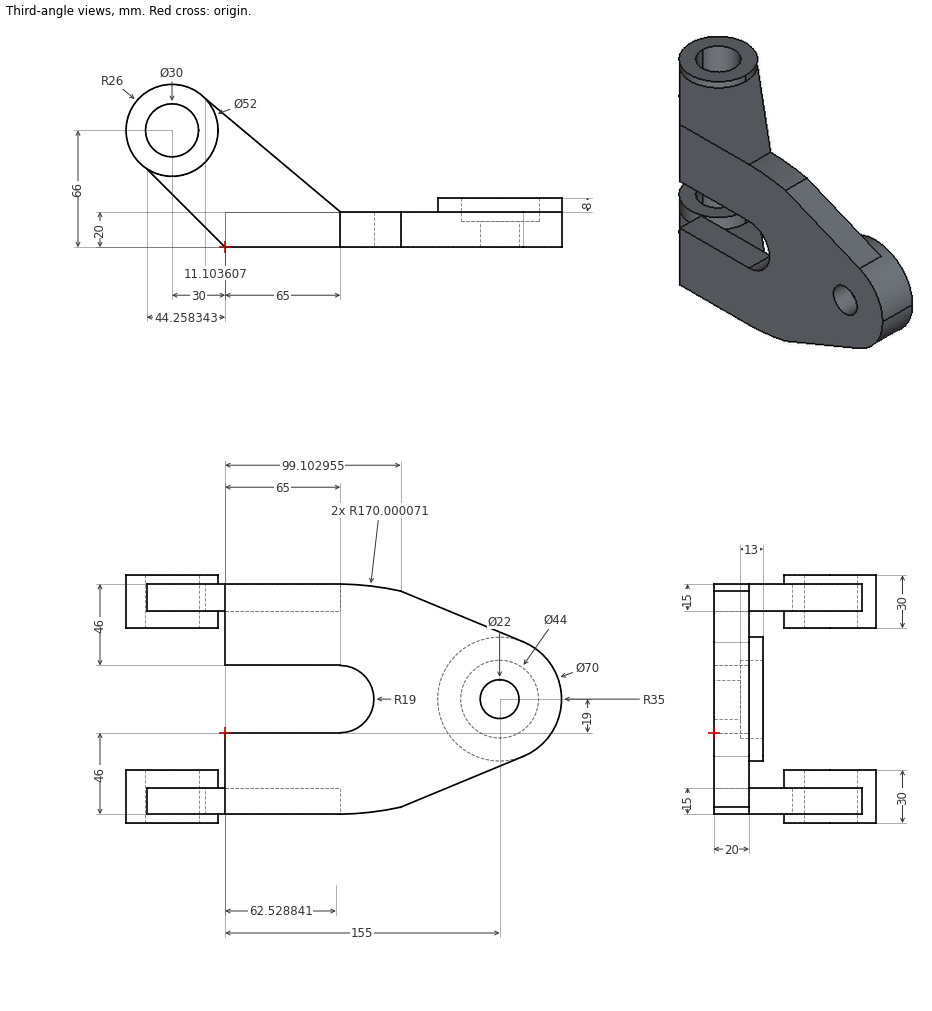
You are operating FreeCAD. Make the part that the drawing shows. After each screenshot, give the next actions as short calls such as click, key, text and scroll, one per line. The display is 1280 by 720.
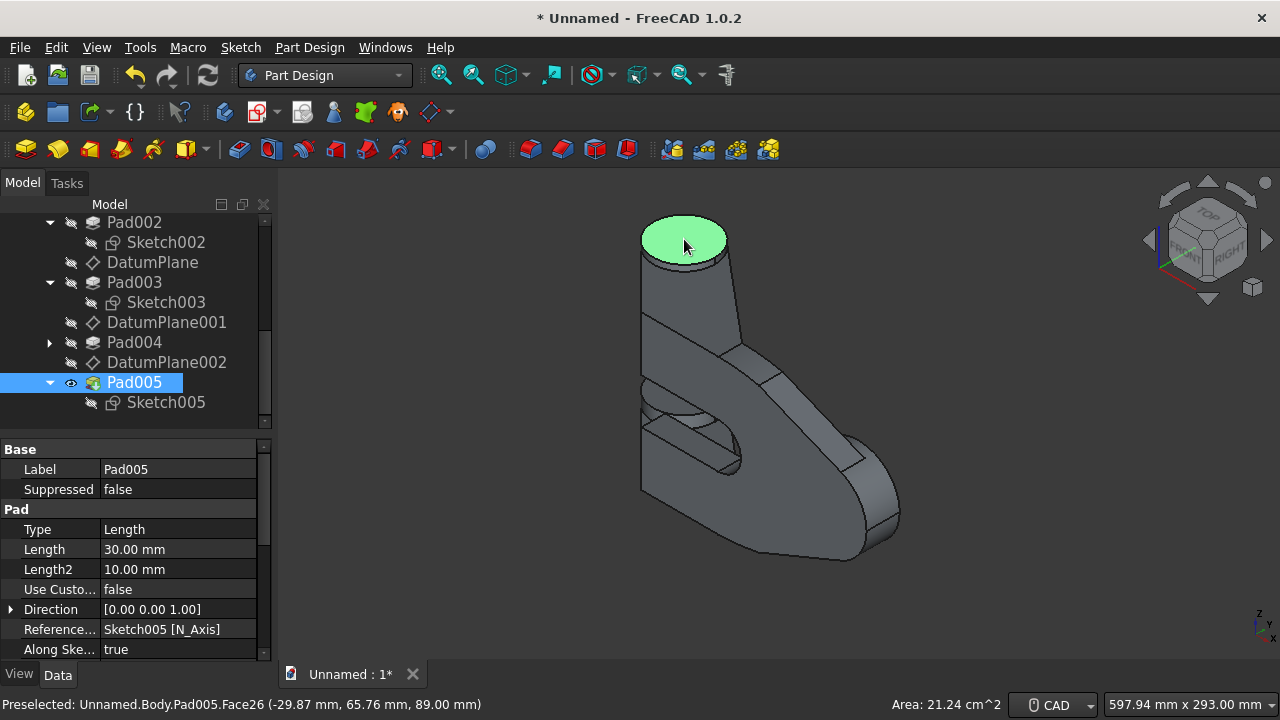
click(258, 112)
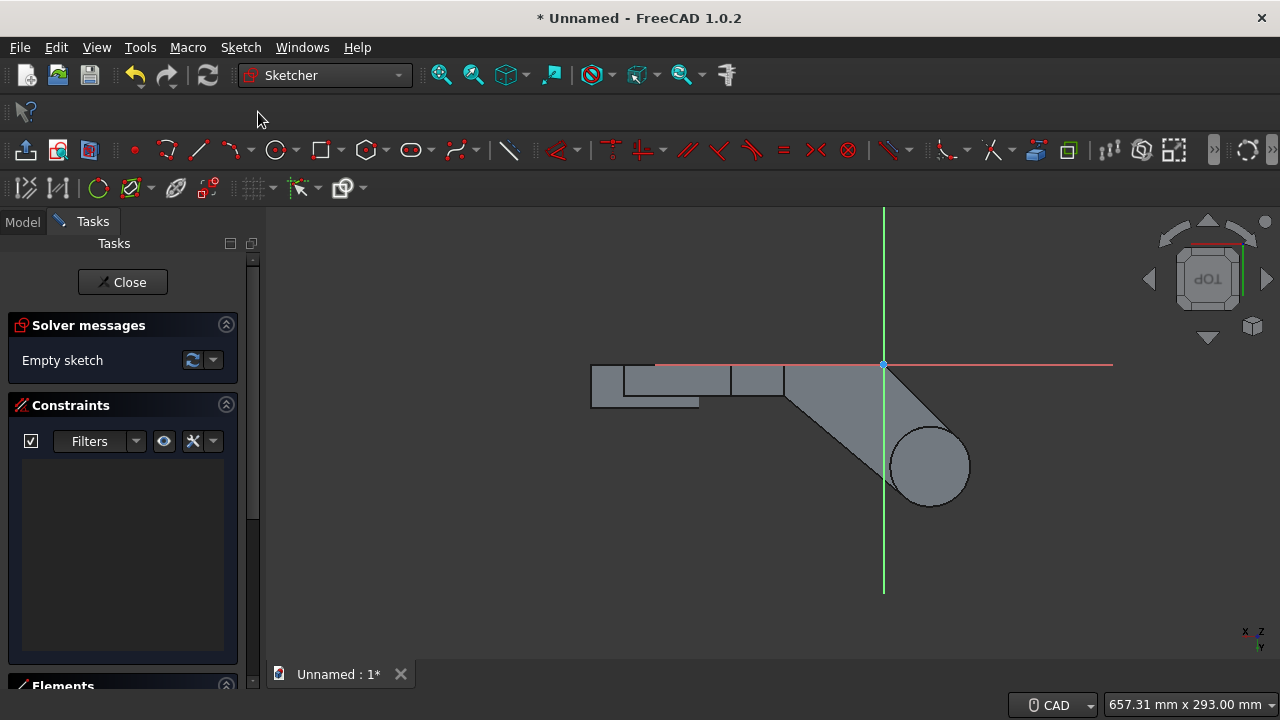
scroll(975, 473, up, 9)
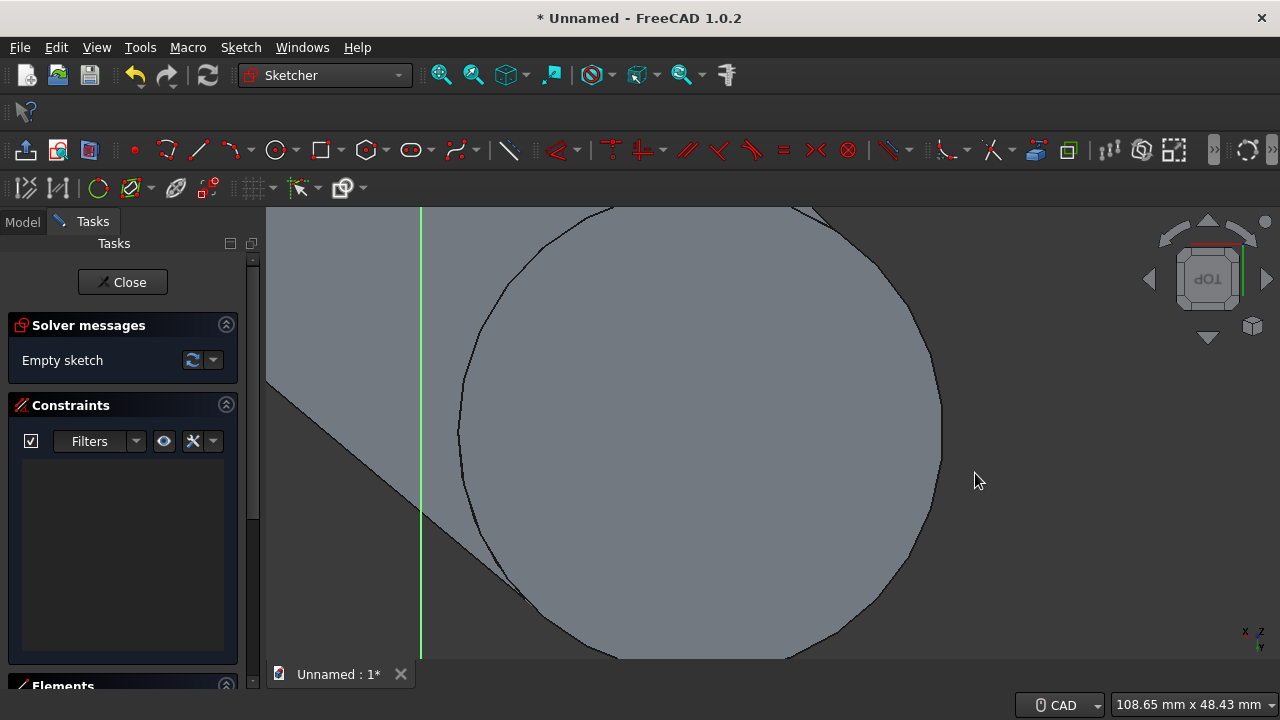
key(g)
key(c)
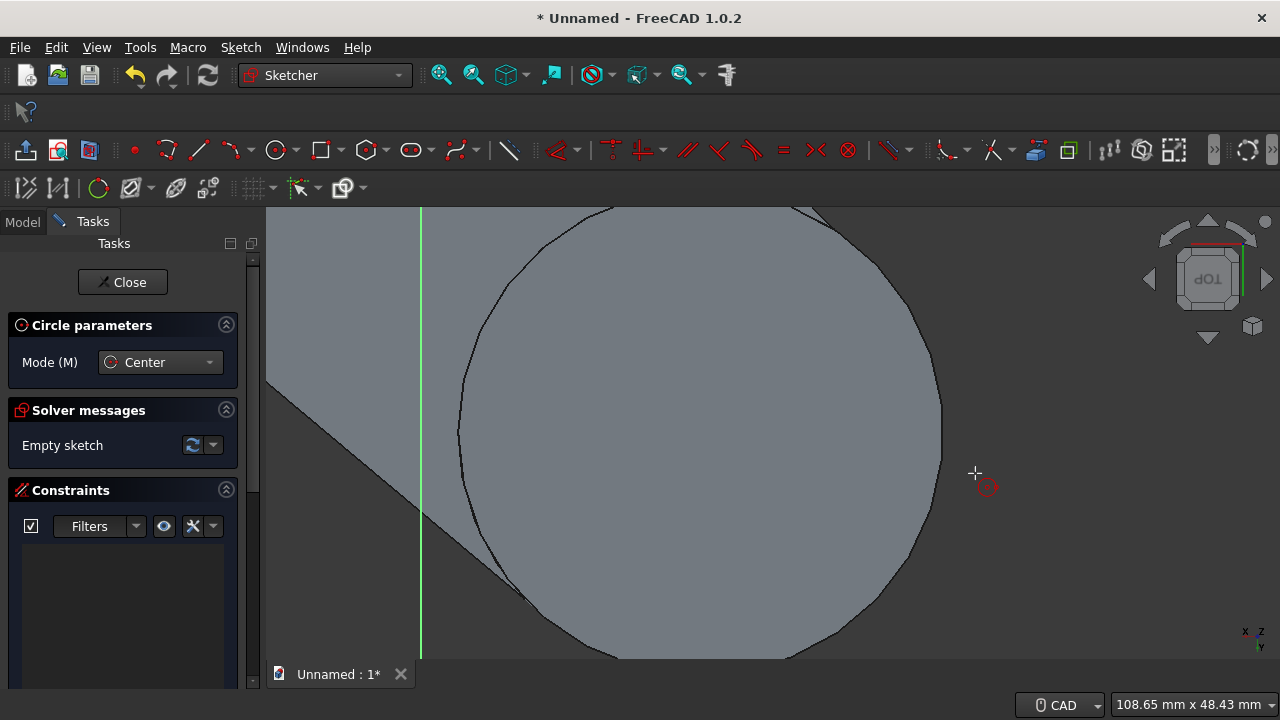
click(701, 432)
move(800, 333)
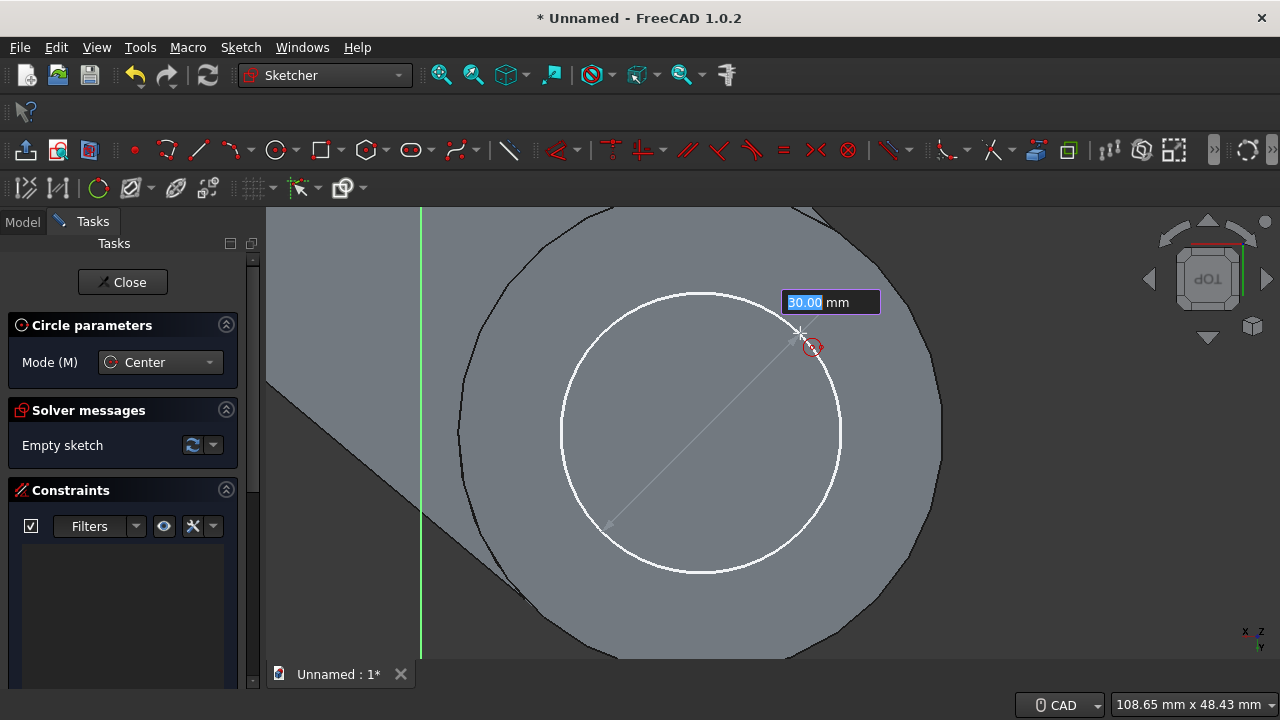
text(30)
key(Return)
key(Escape)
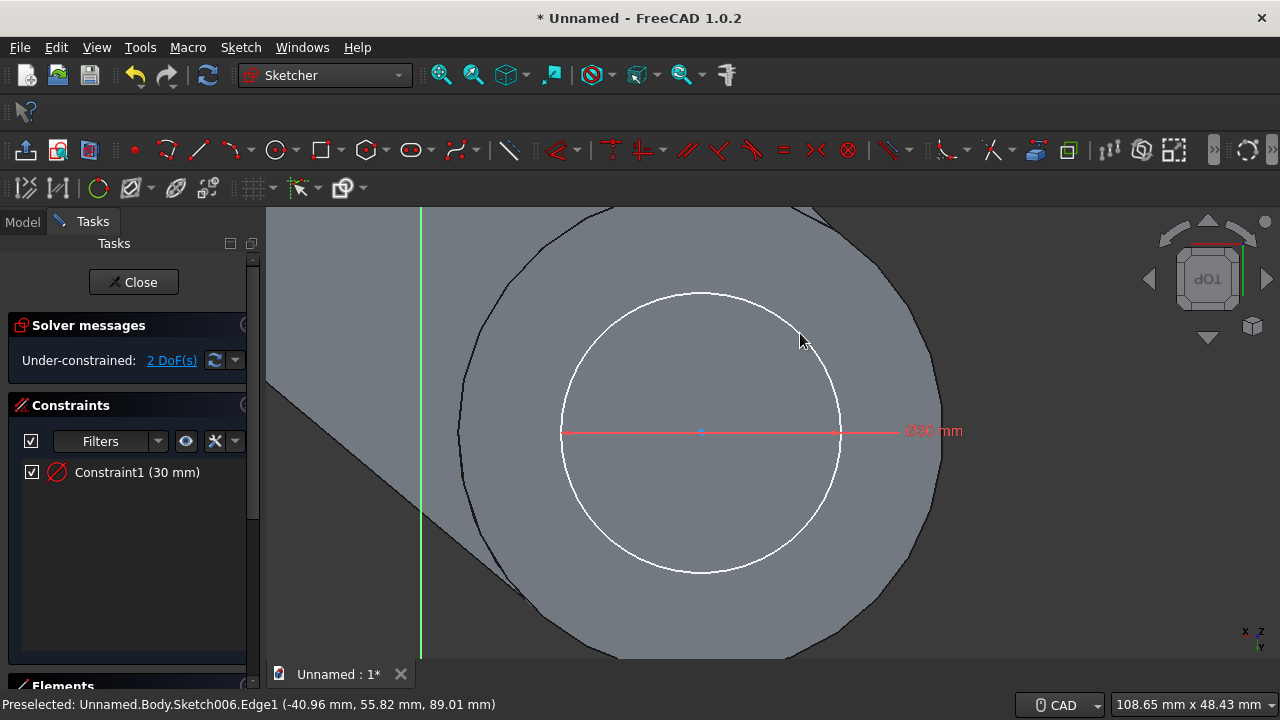
key(d)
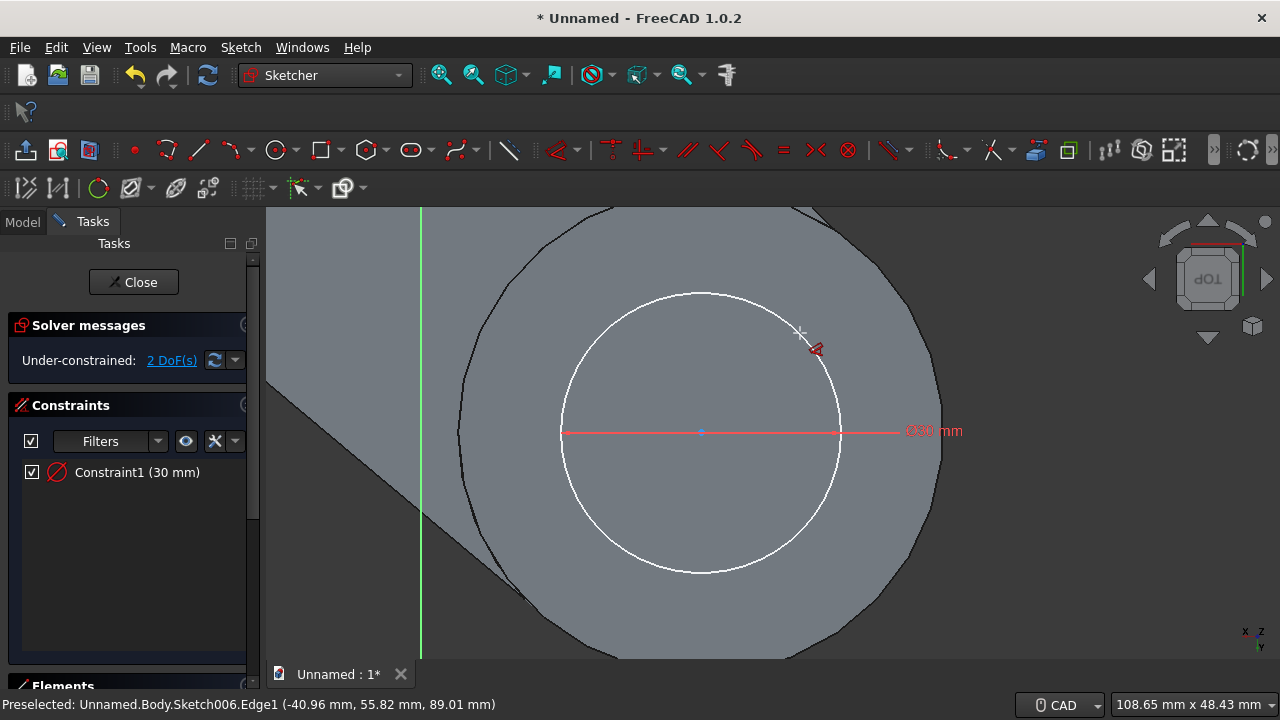
click(701, 433)
click(496, 467)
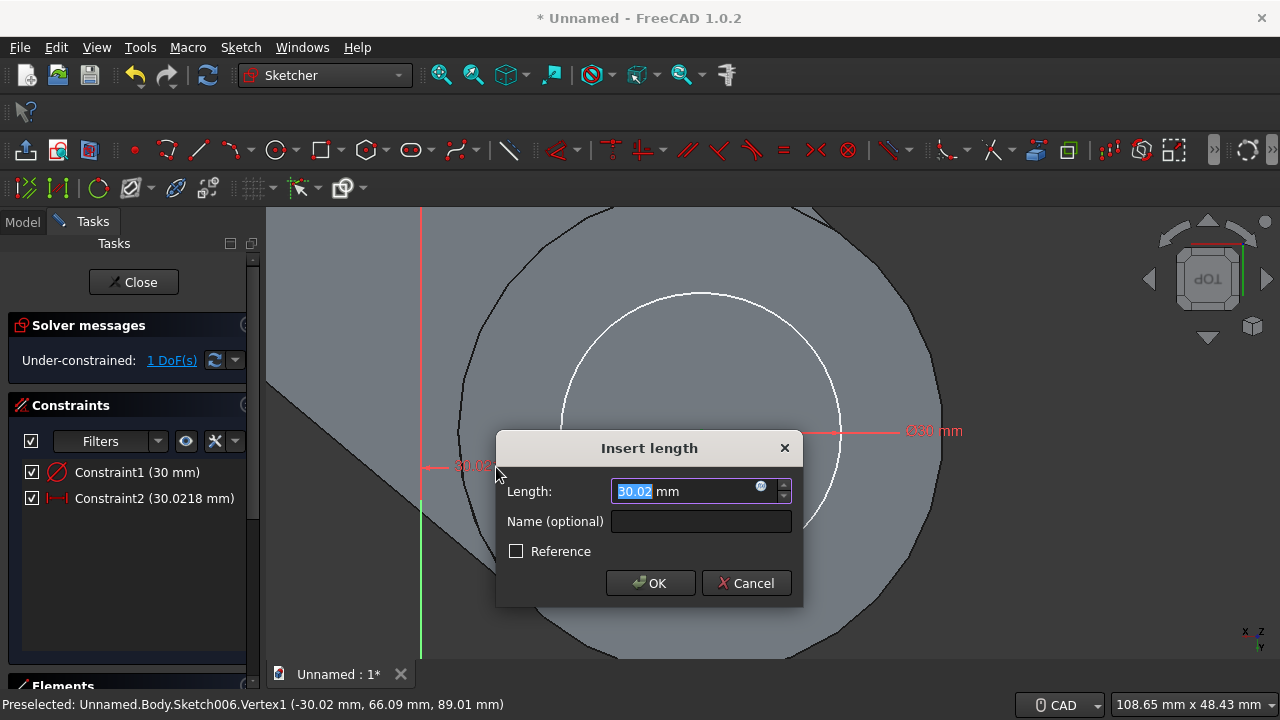
text(30)
key(Return)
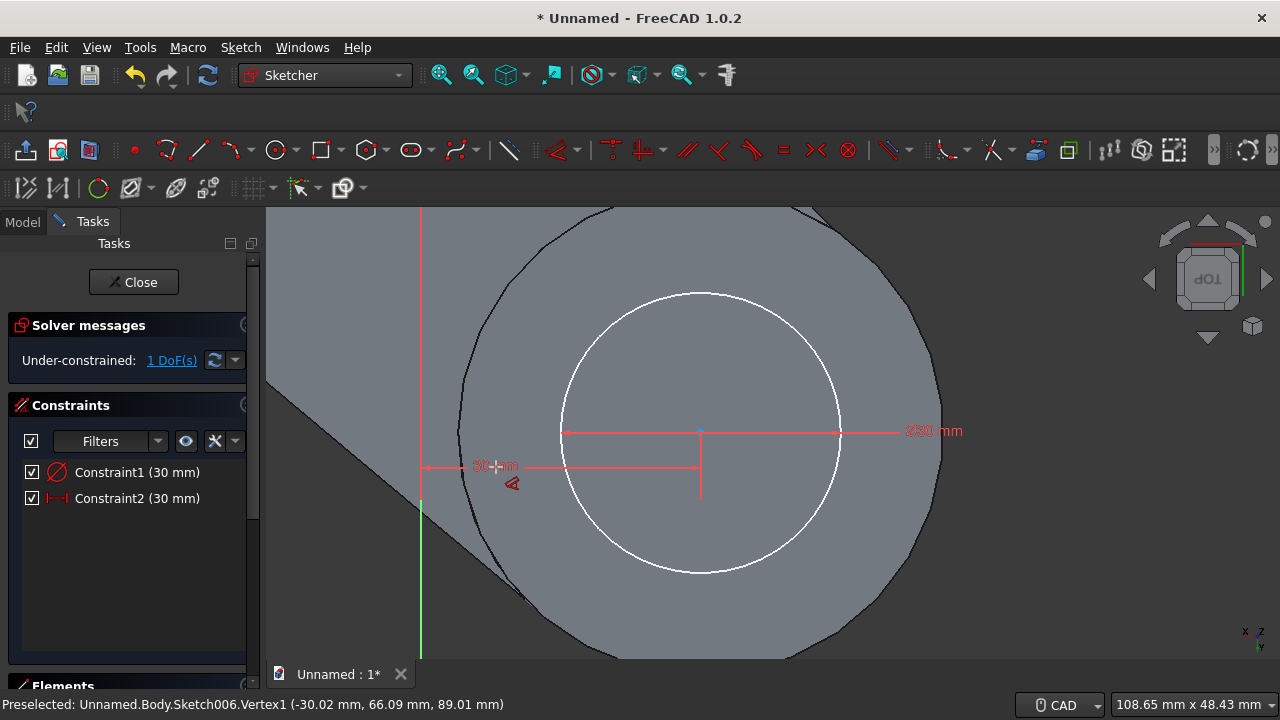
click(701, 433)
click(387, 334)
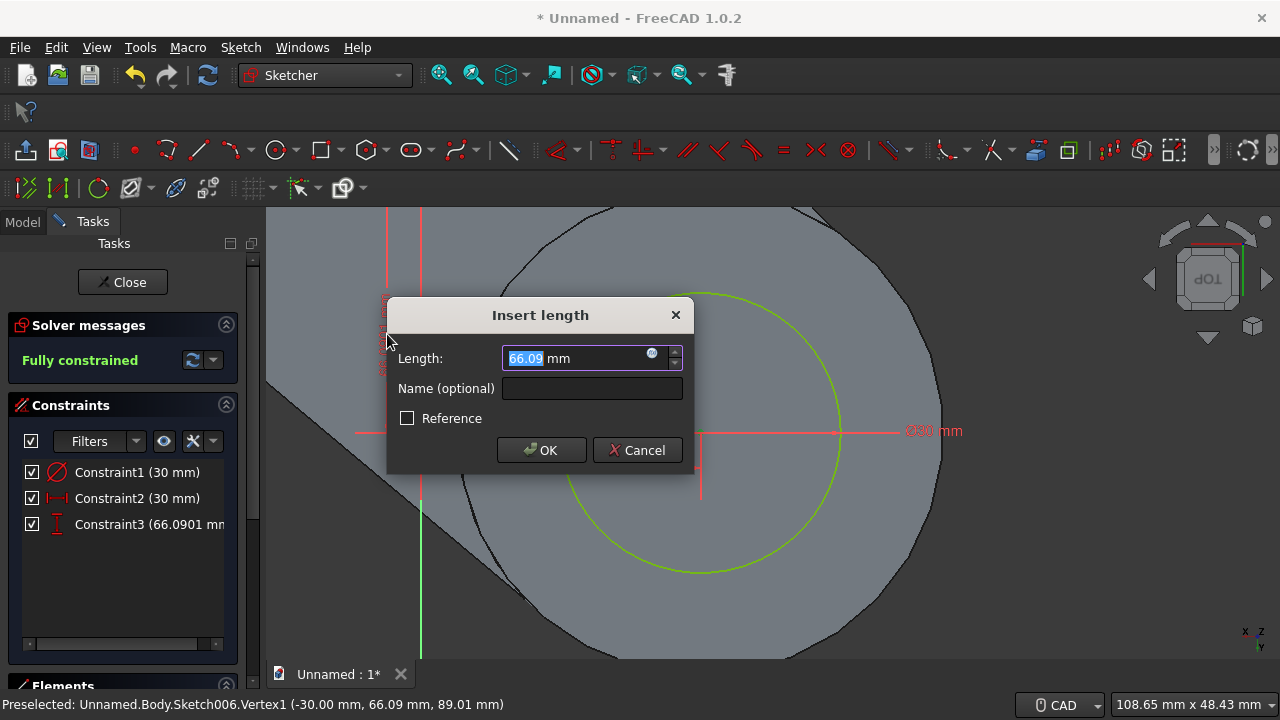
text(66)
key(Return)
key(Escape)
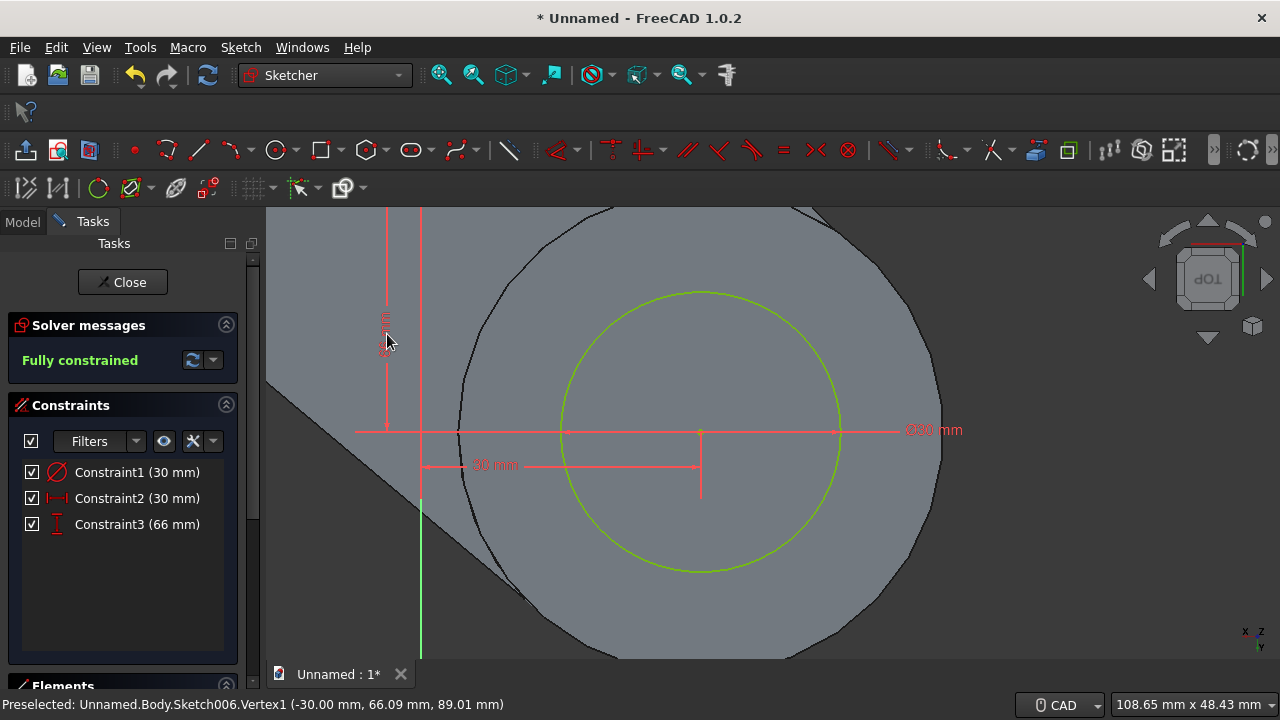
click(123, 282)